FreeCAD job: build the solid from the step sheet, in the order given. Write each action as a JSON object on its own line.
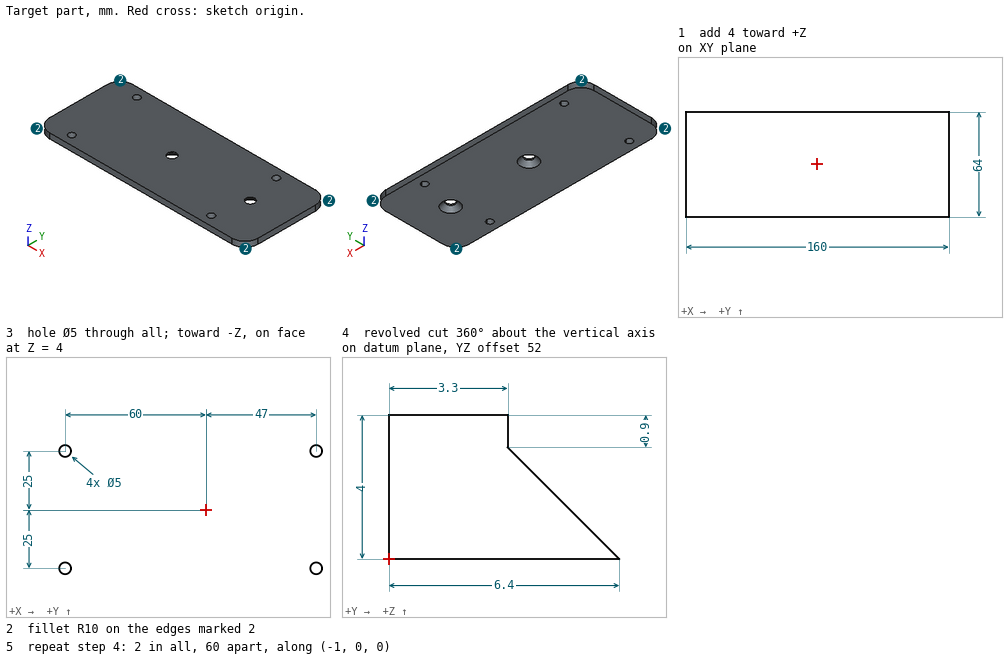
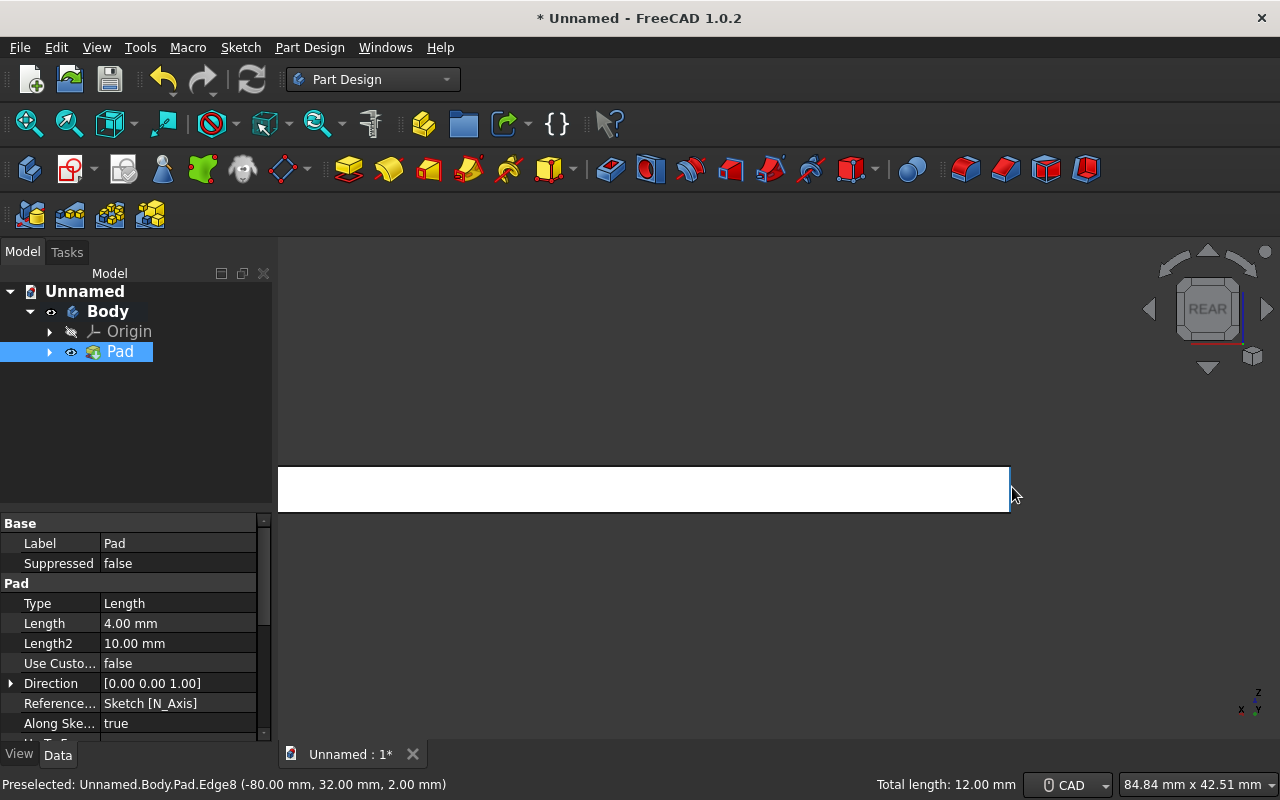
{"action": "left_click", "coordinate": [1010, 489], "text": "ctrl"}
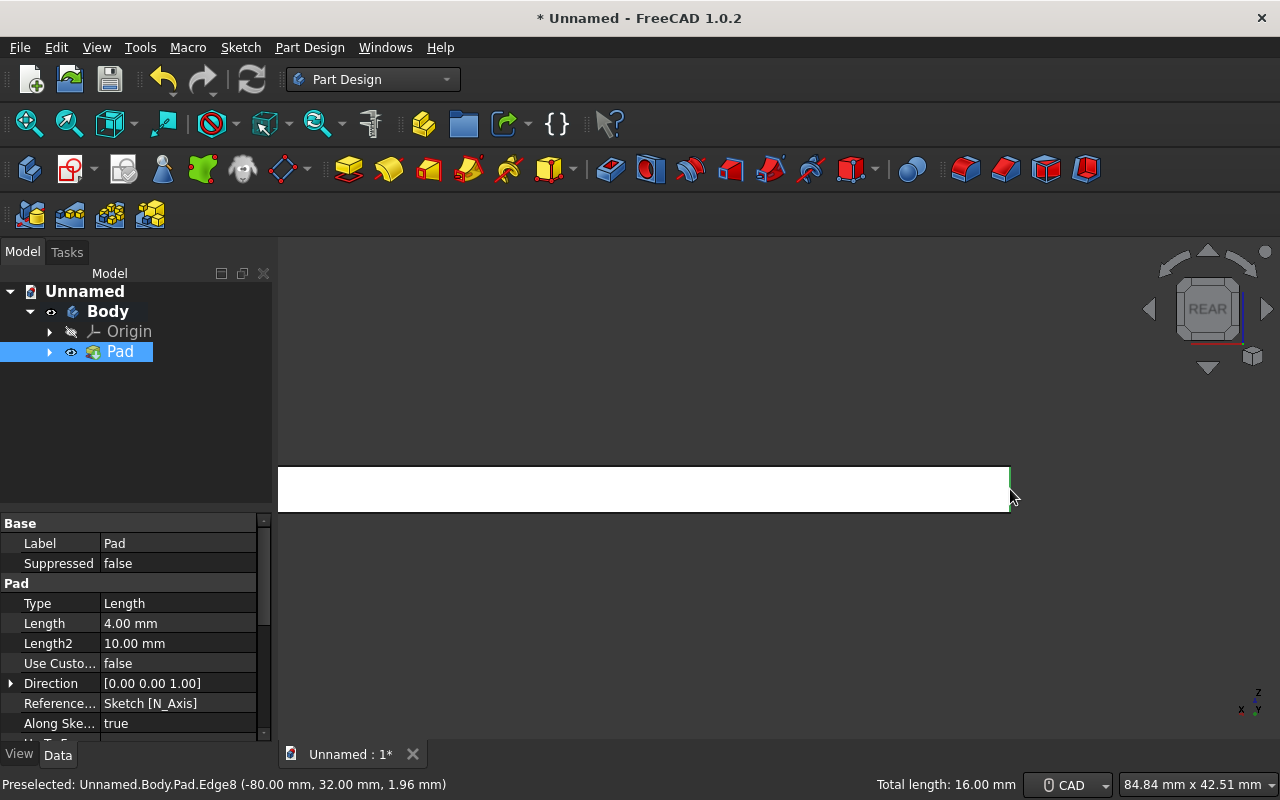
{"action": "left_click", "coordinate": [966, 170]}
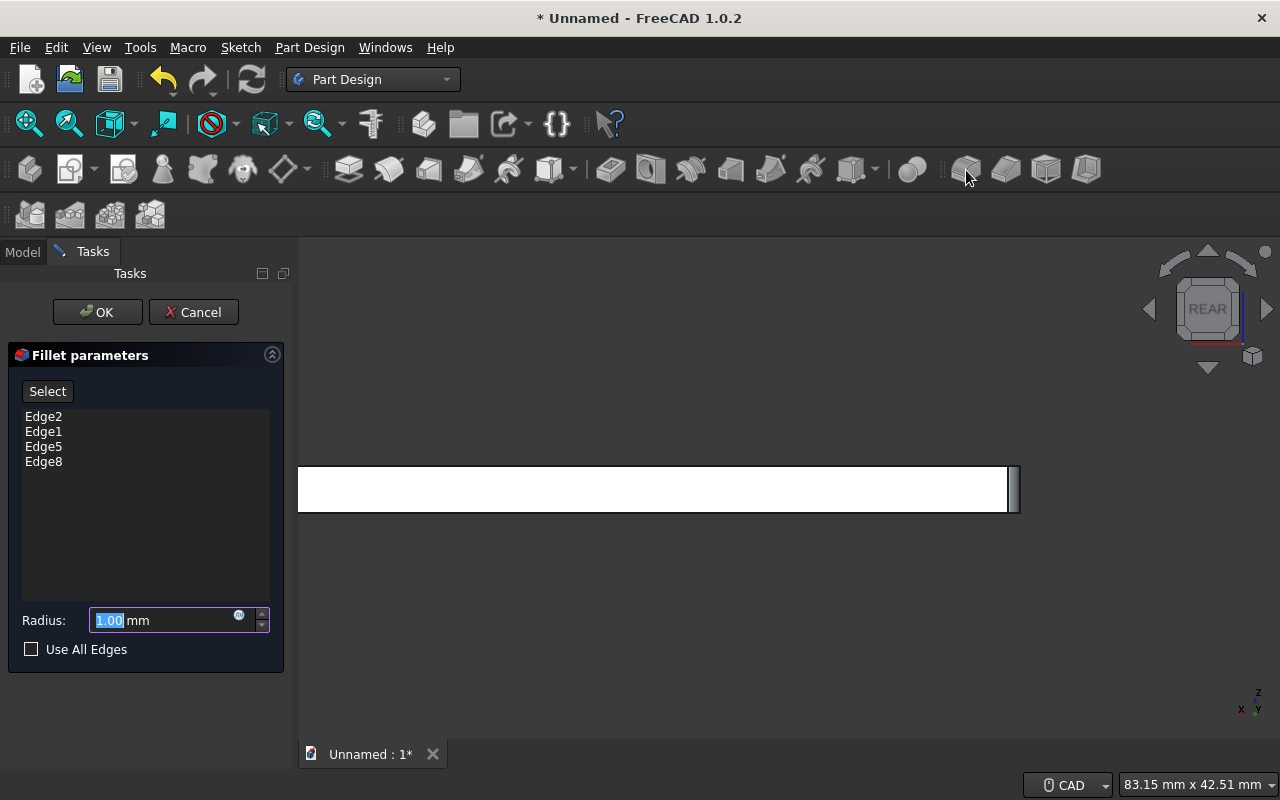
{"action": "type", "text": "10"}
{"action": "key", "text": "Tab"}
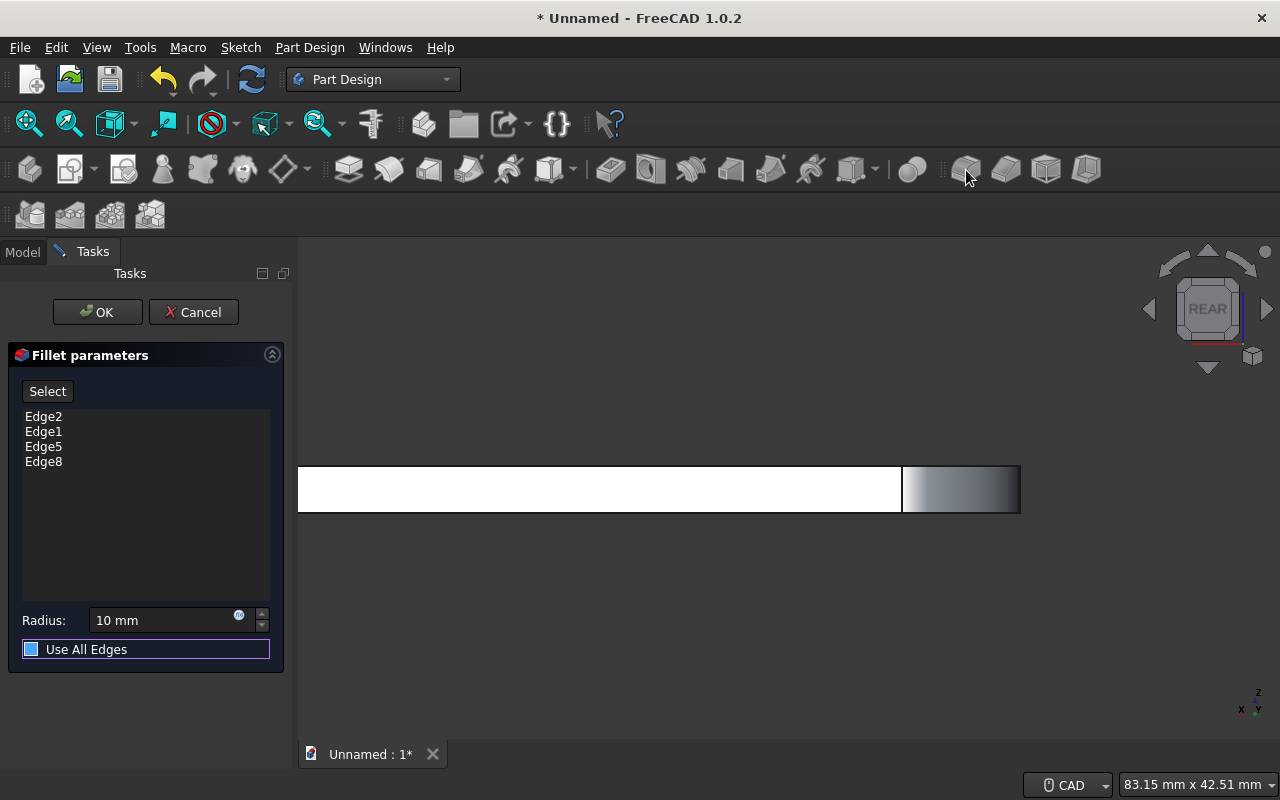
{"action": "left_click", "coordinate": [98, 312]}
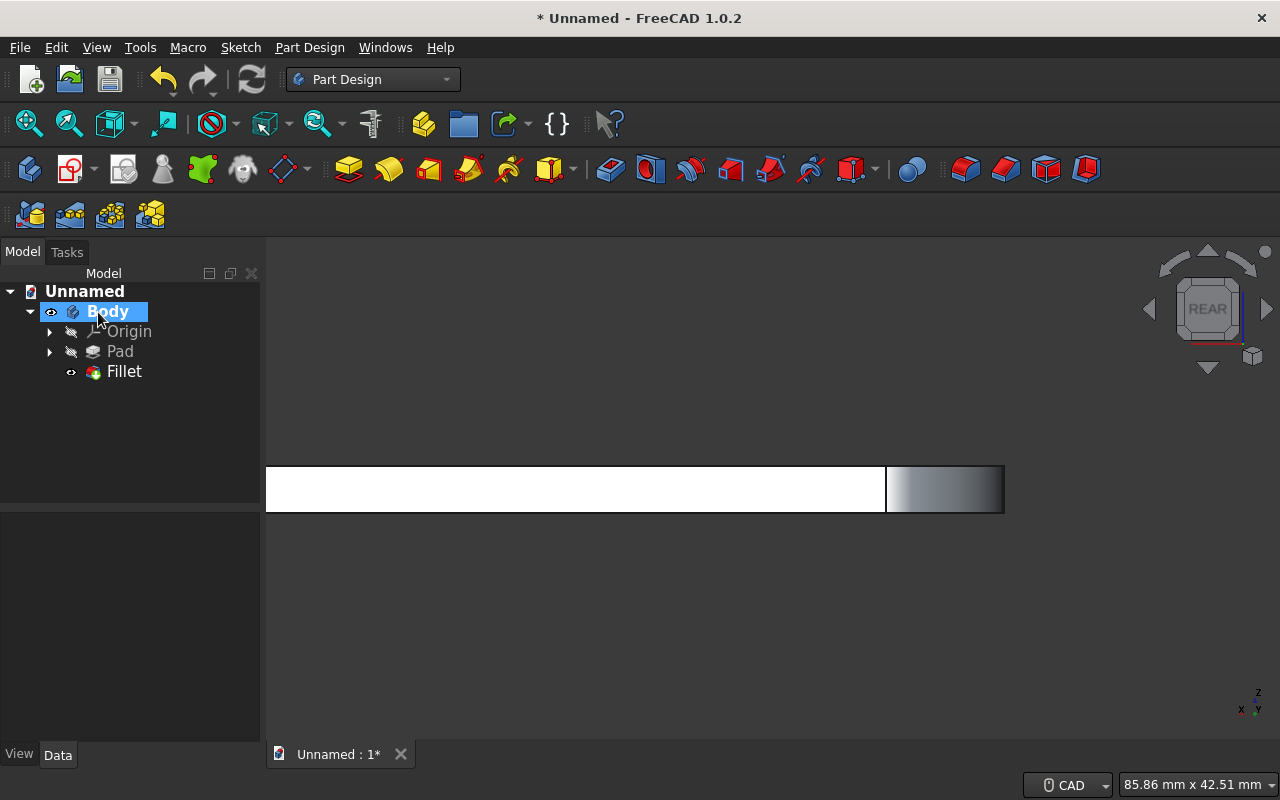
{"action": "left_click", "coordinate": [30, 124]}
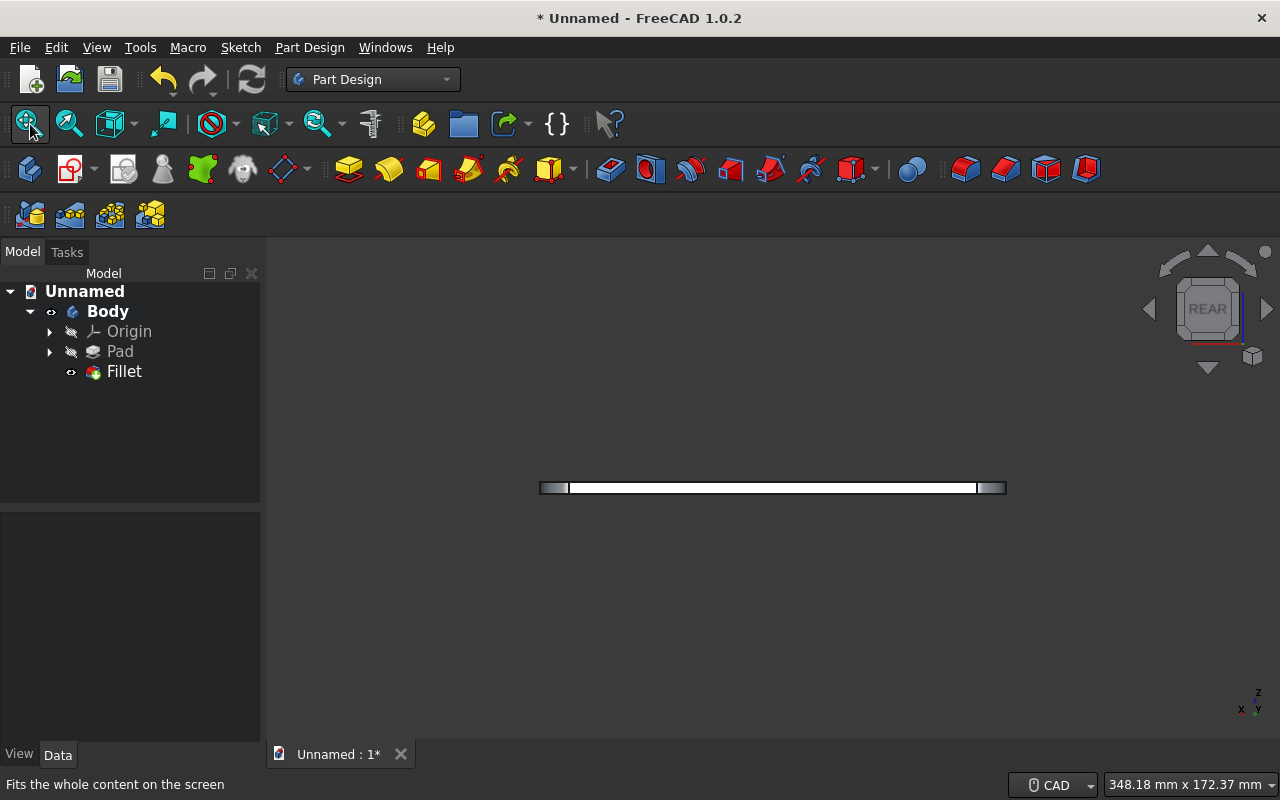
{"action": "key", "text": "0"}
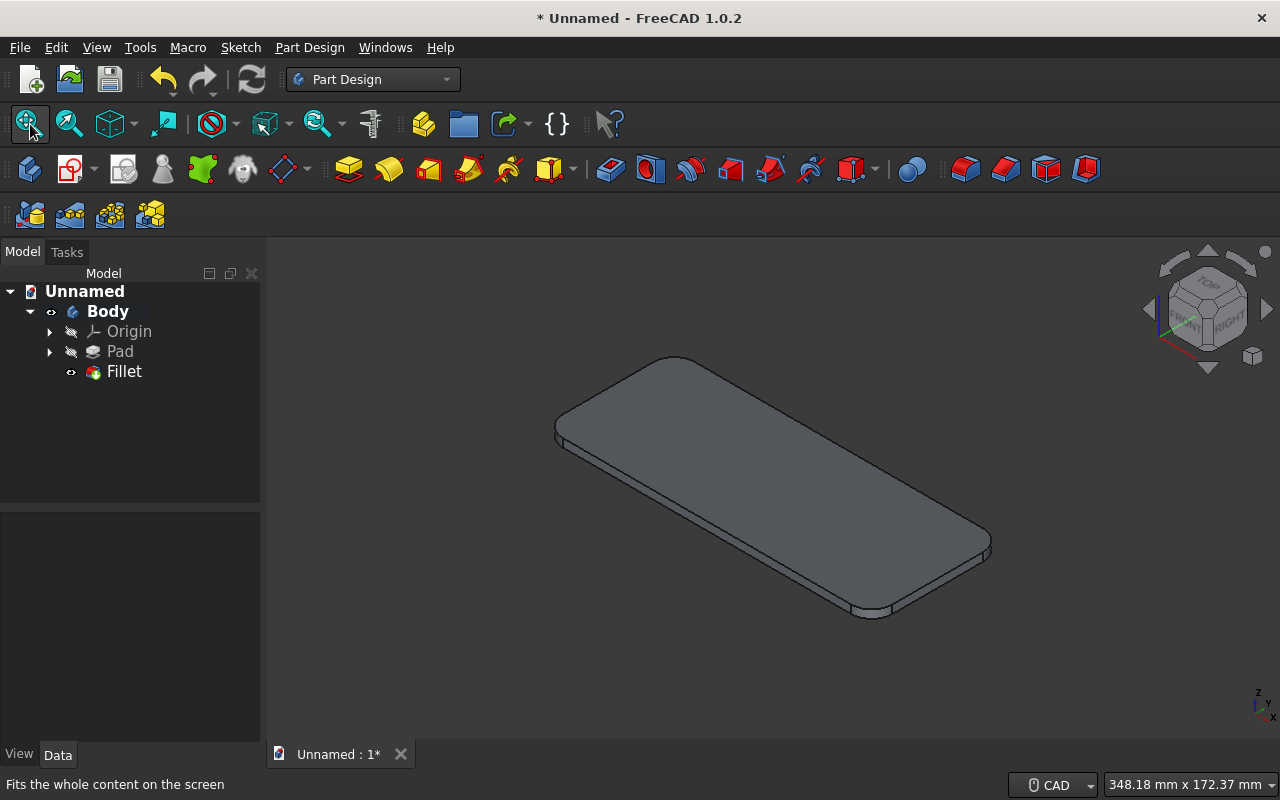
{"action": "left_click", "coordinate": [867, 537]}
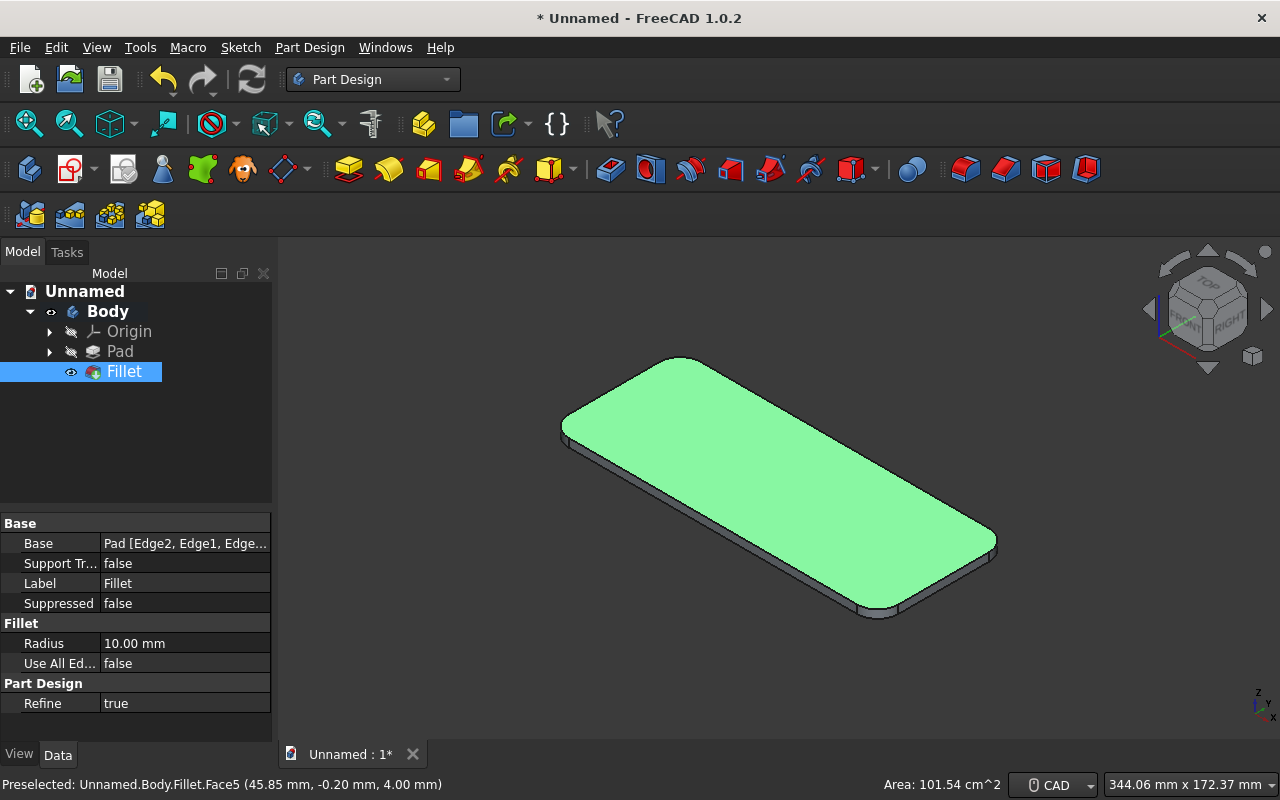
{"action": "left_click", "coordinate": [70, 170]}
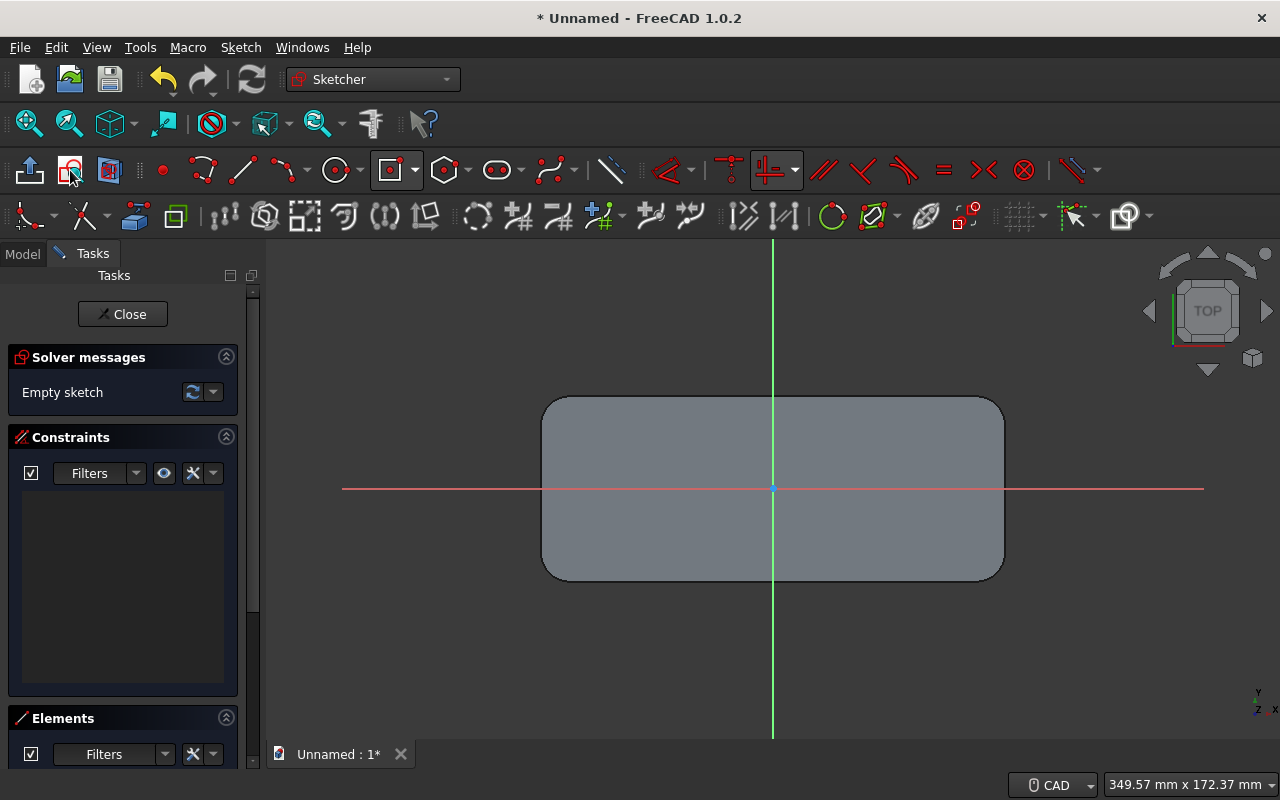
{"action": "scroll", "coordinate": [815, 489], "scroll_direction": "up", "scroll_amount": 3}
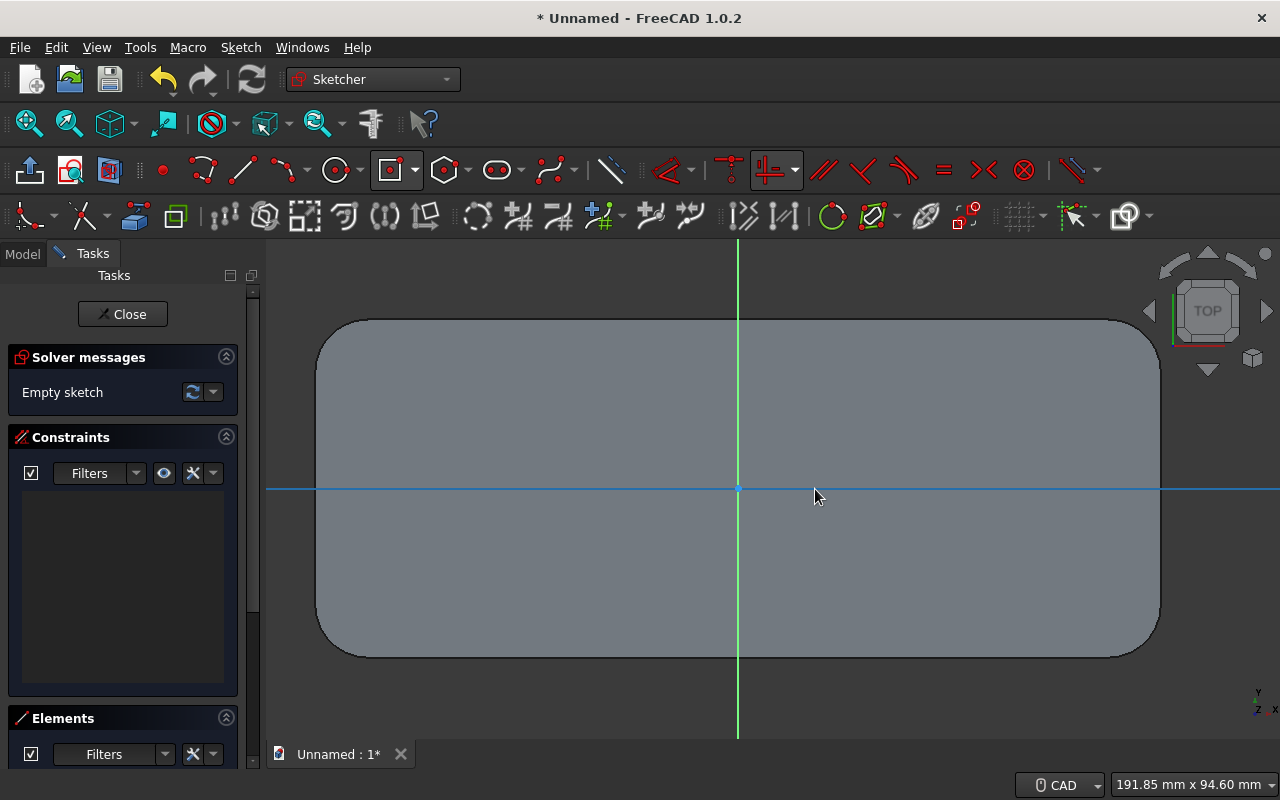
{"action": "left_click", "coordinate": [336, 170]}